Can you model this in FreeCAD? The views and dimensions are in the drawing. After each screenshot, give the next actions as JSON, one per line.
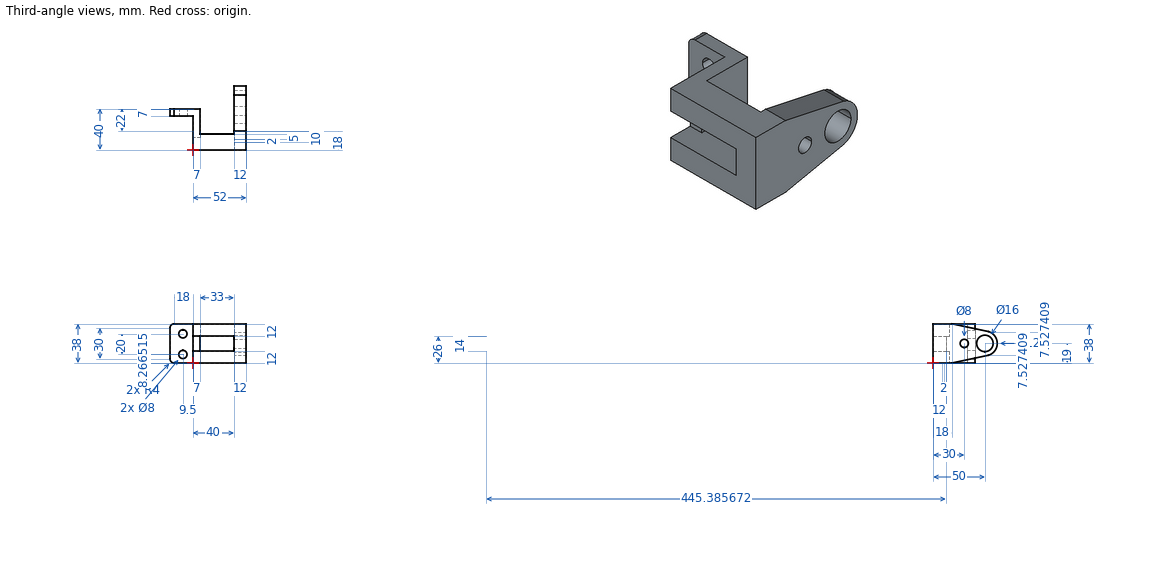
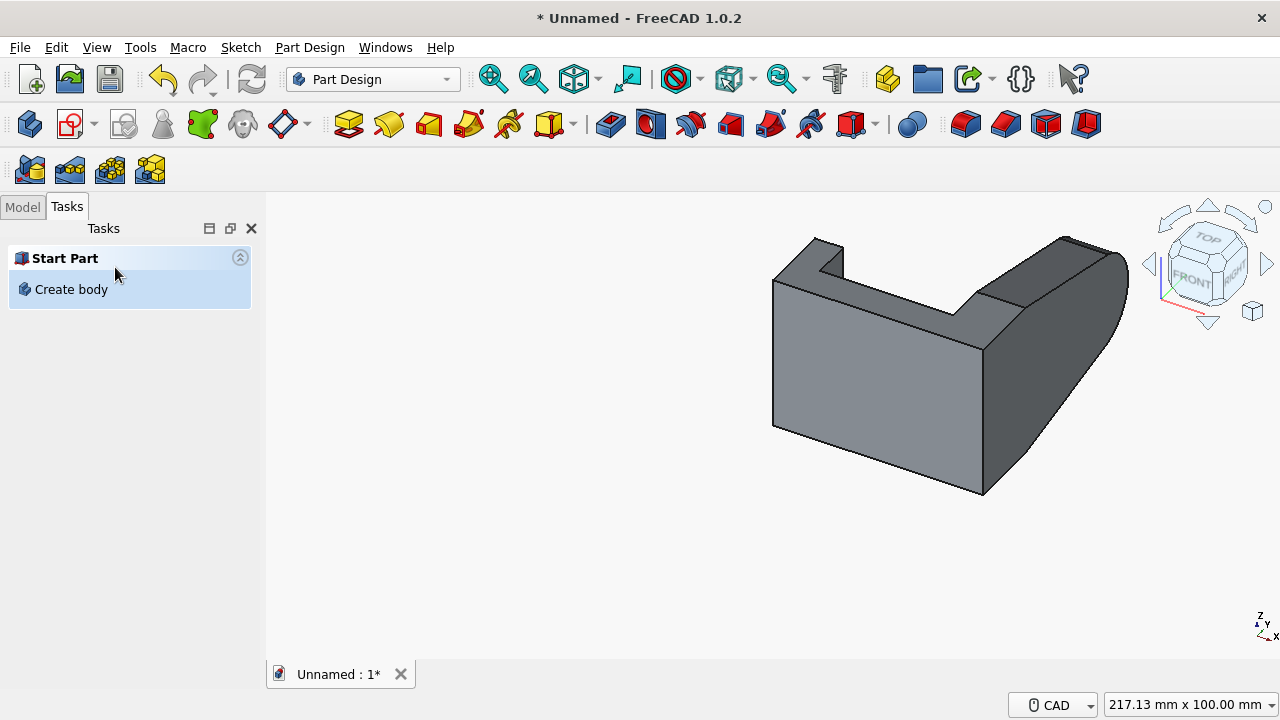
{"action": "left_click", "coordinate": [494, 80]}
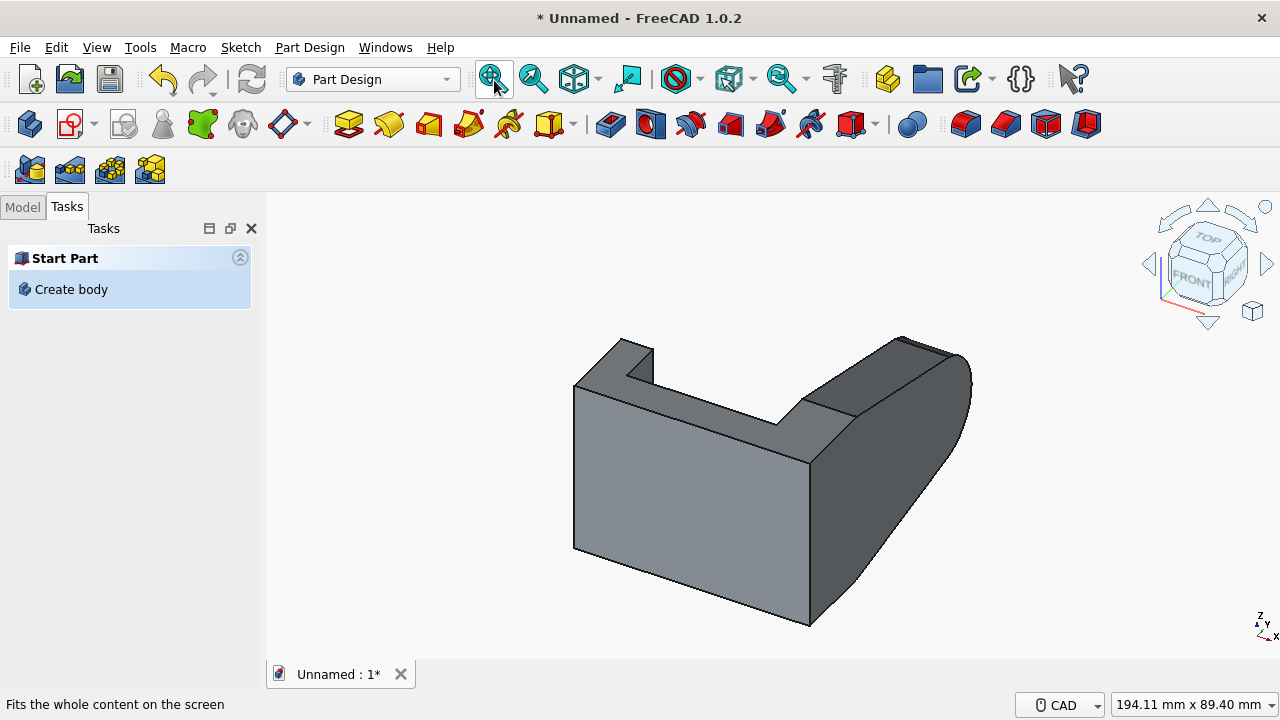
{"action": "left_click", "coordinate": [70, 124]}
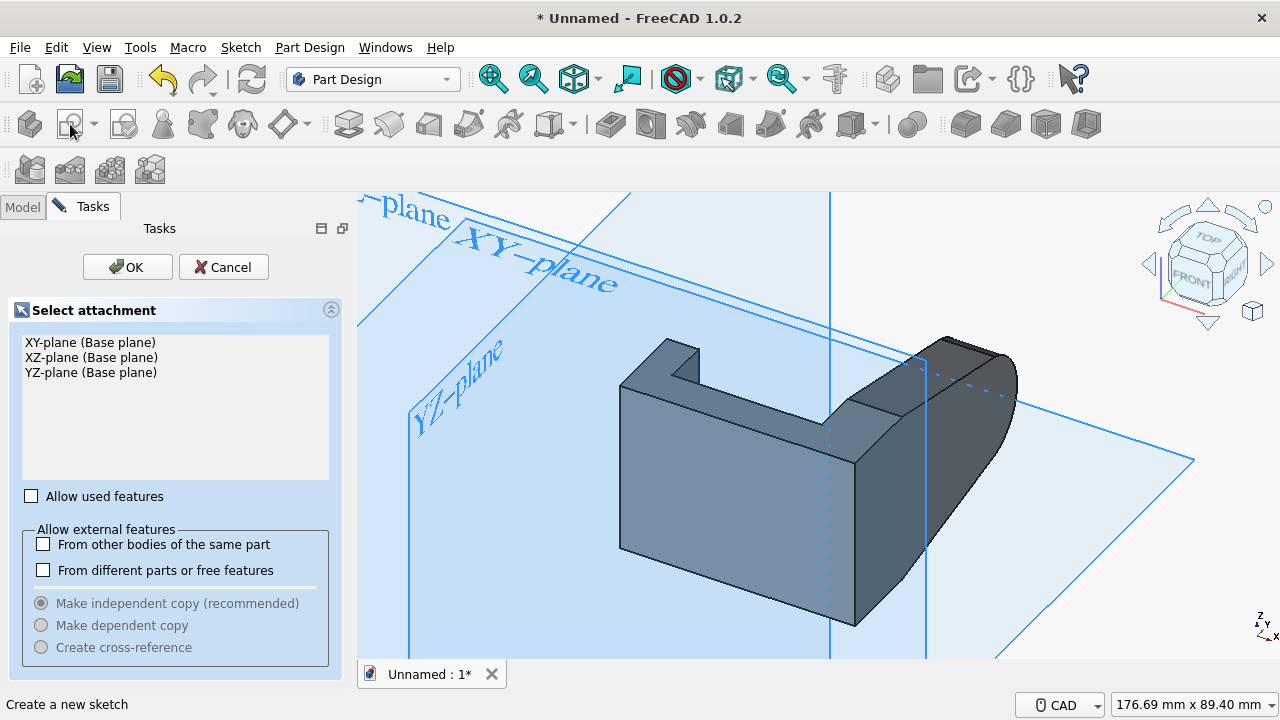
{"action": "left_click", "coordinate": [82, 372]}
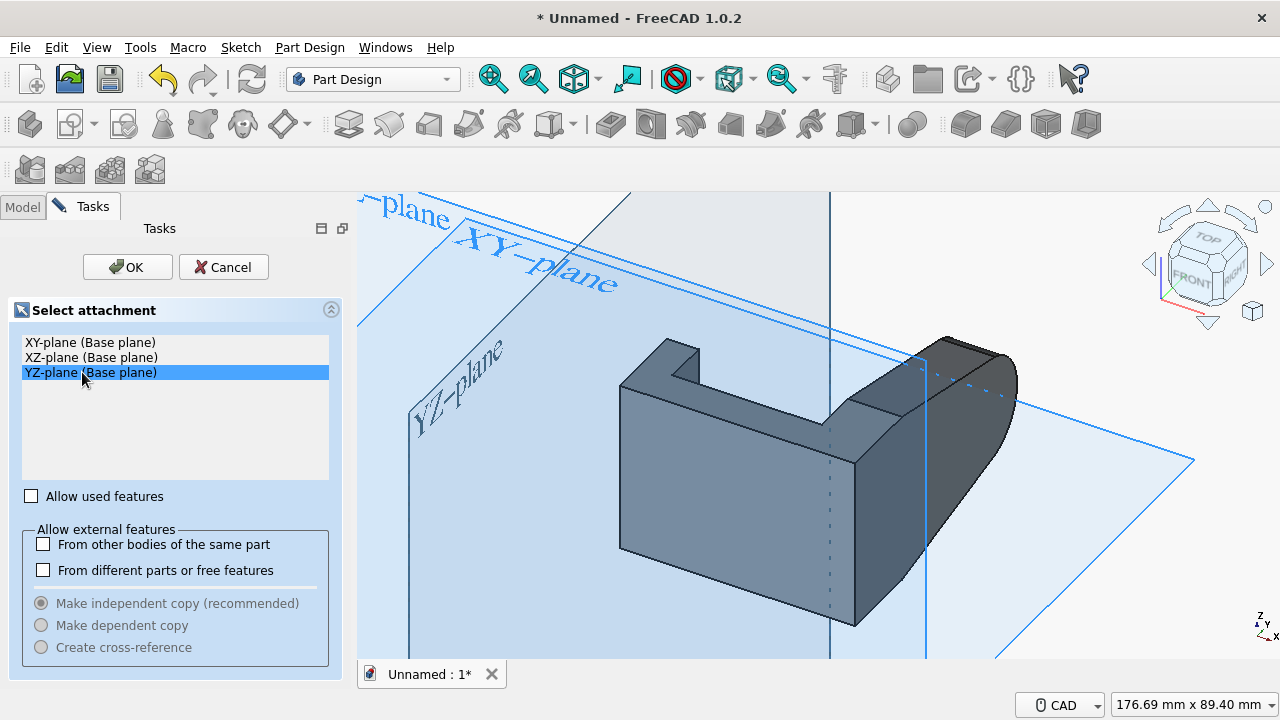
{"action": "left_click", "coordinate": [128, 267]}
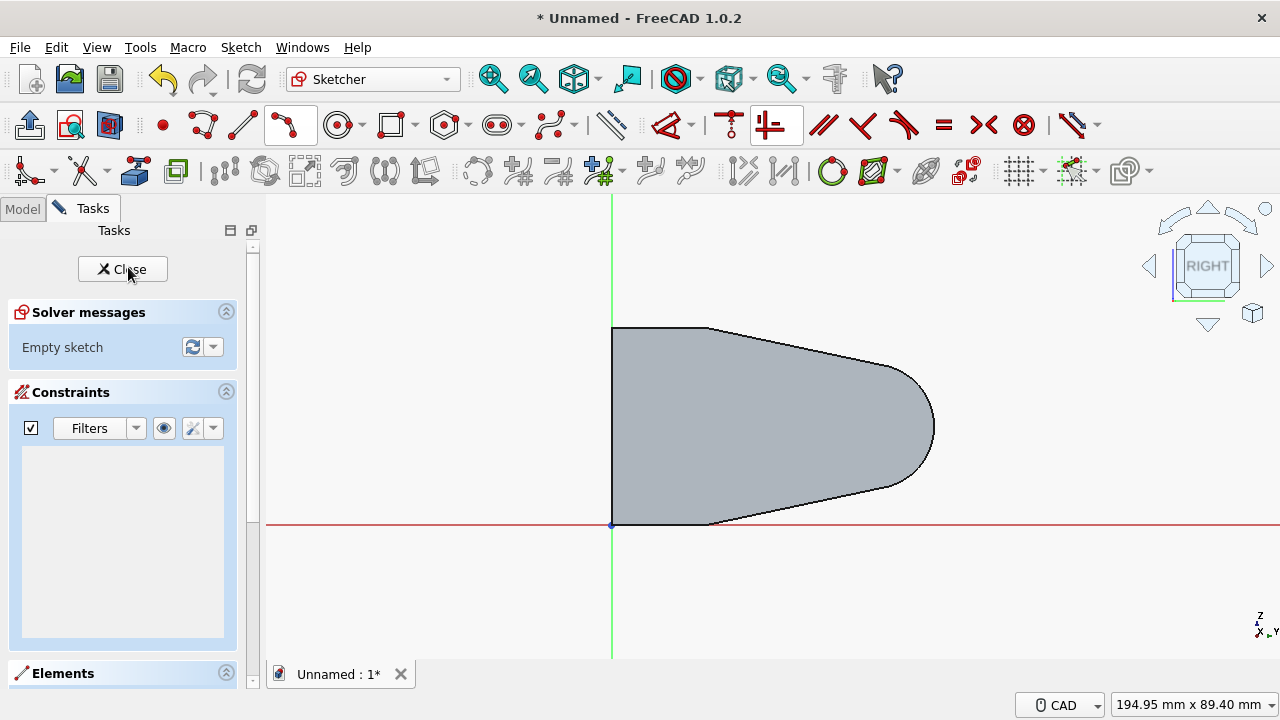
{"action": "left_click", "coordinate": [110, 126]}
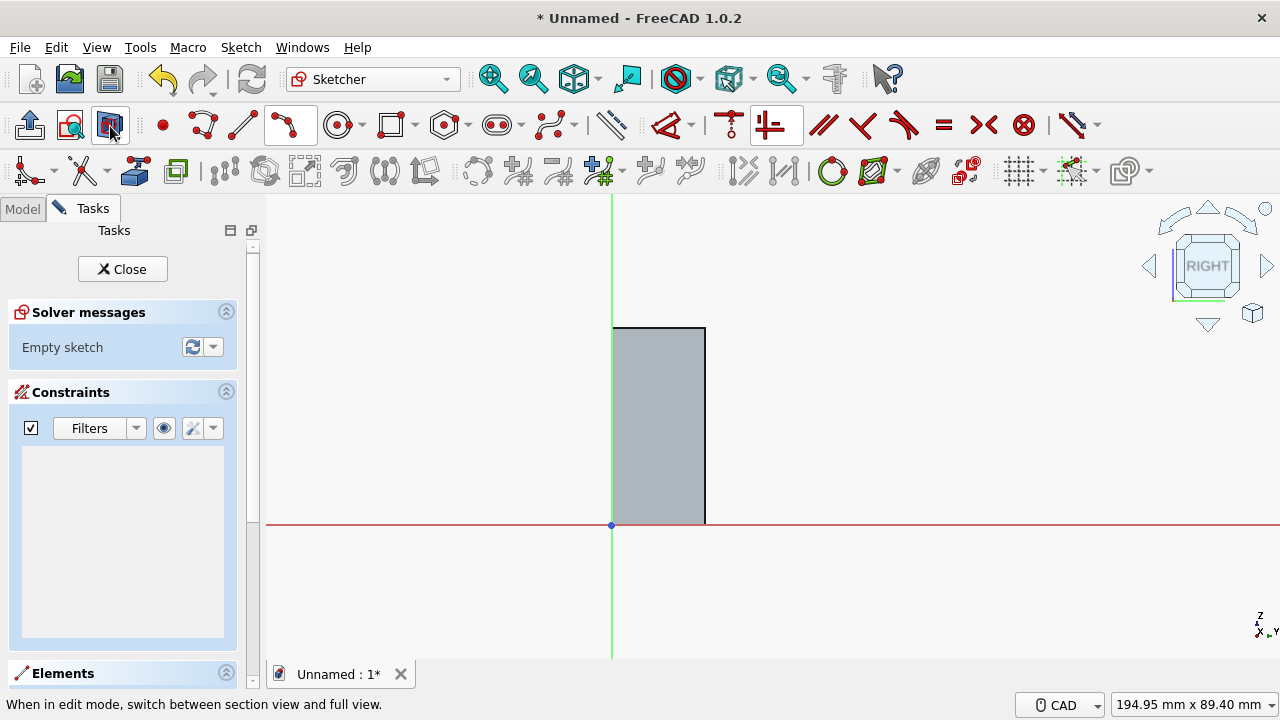
{"action": "scroll", "coordinate": [1094, 416], "scroll_direction": "down", "scroll_amount": 7}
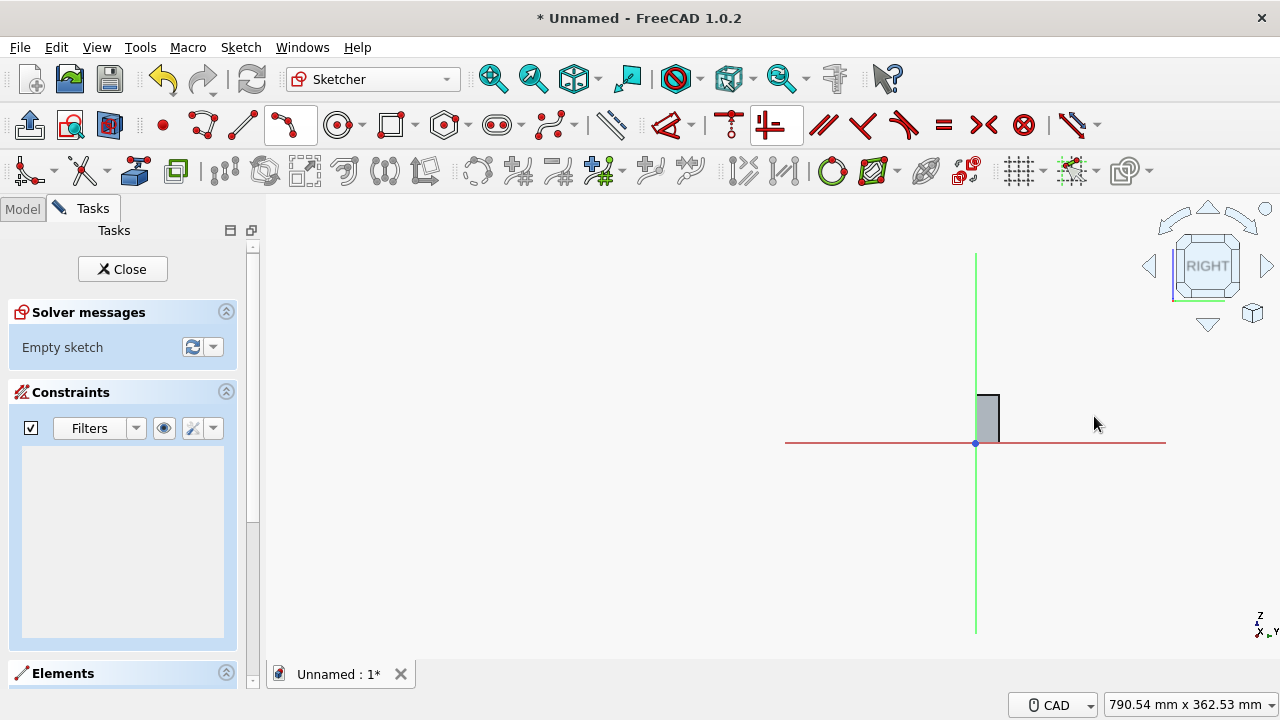
{"action": "left_click", "coordinate": [392, 126]}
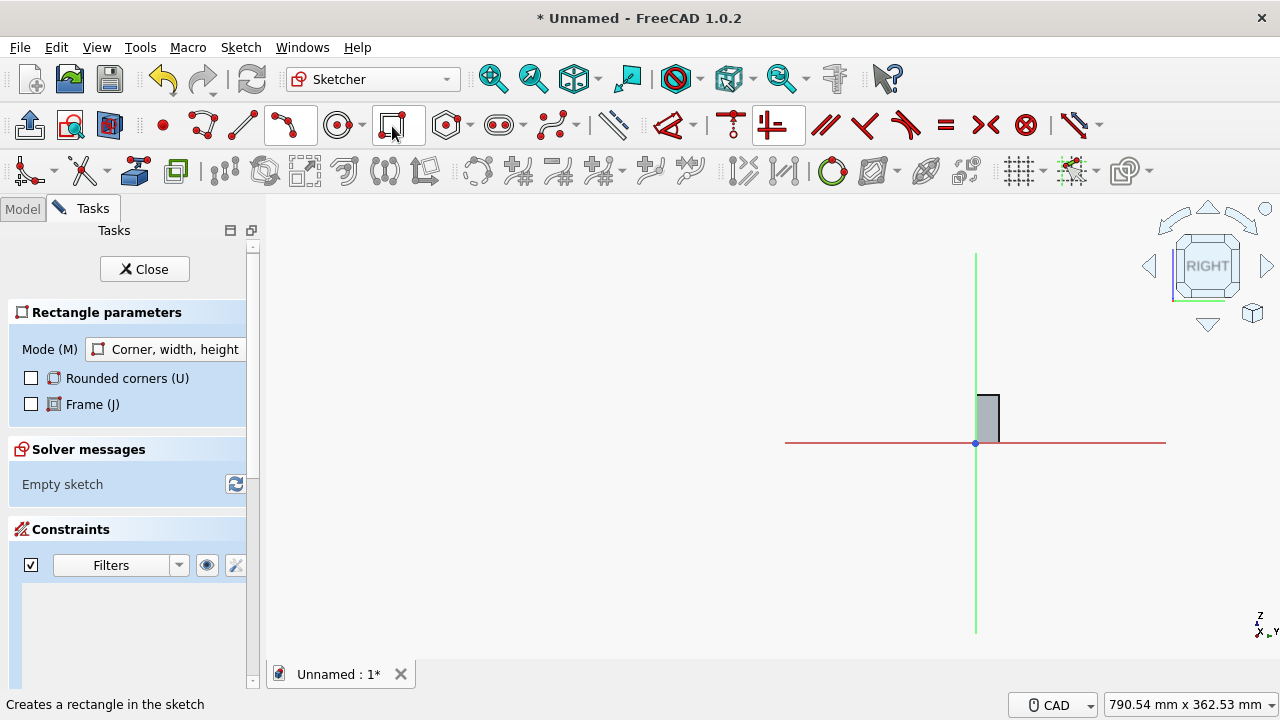
{"action": "left_click", "coordinate": [420, 410]}
{"action": "left_click", "coordinate": [991, 428]}
{"action": "key", "text": "Escape"}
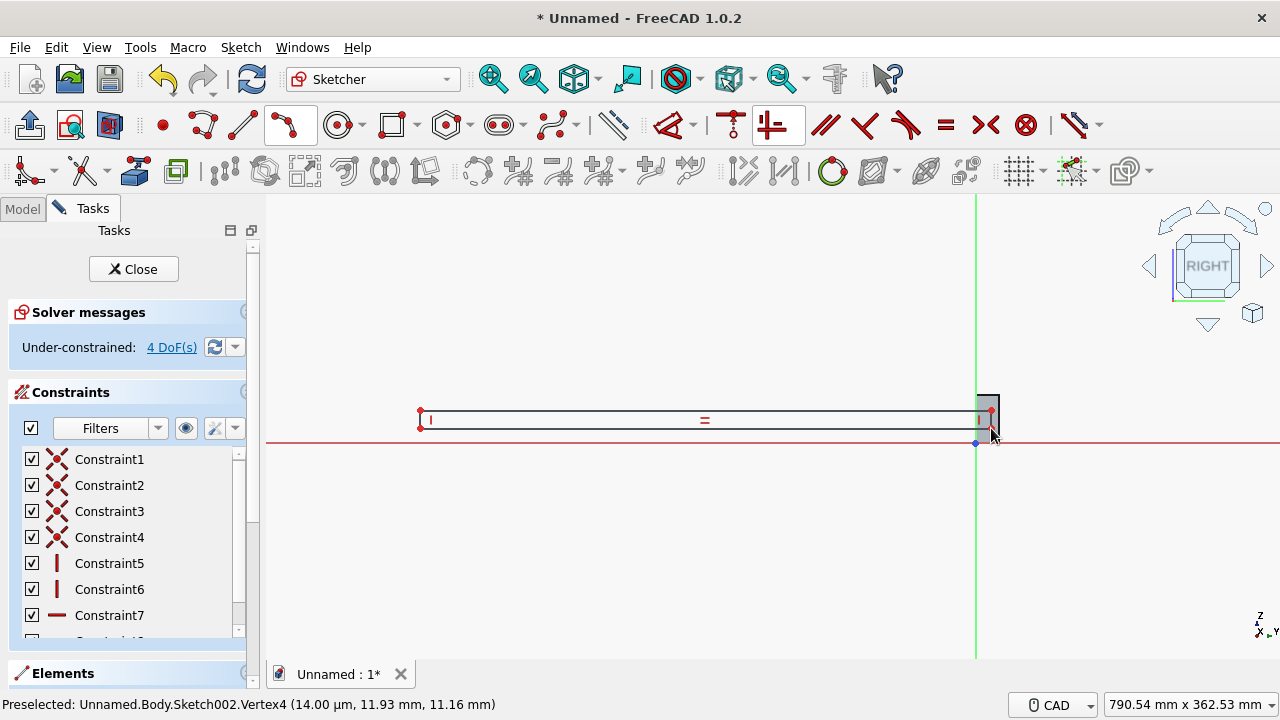
{"action": "left_click", "coordinate": [668, 126]}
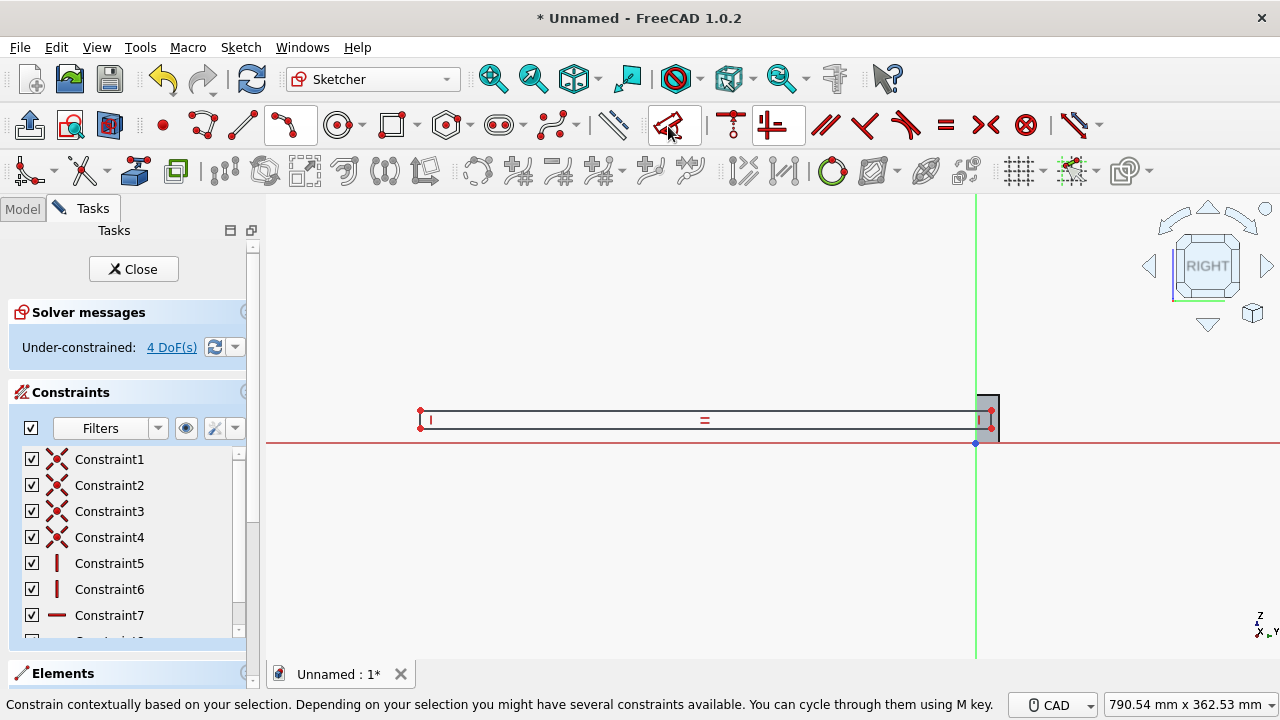
{"action": "scroll", "coordinate": [420, 420], "scroll_direction": "up", "scroll_amount": 4}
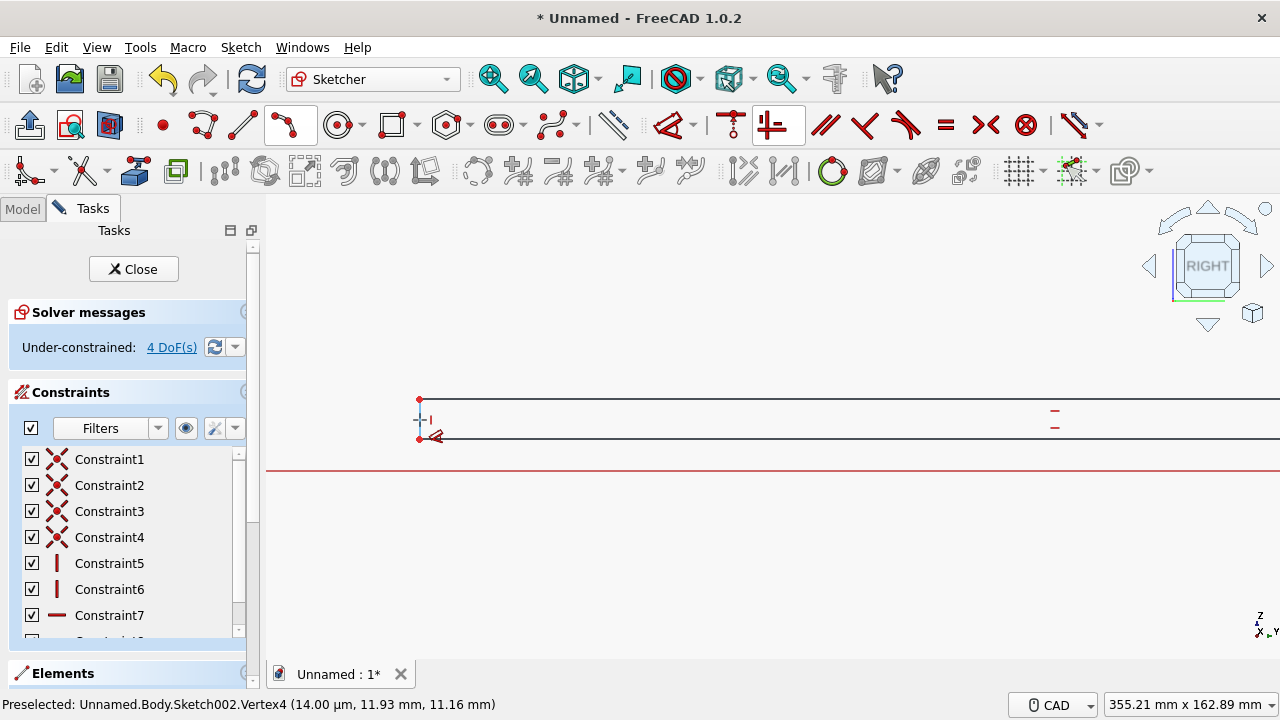
{"action": "left_click", "coordinate": [420, 419]}
{"action": "left_click", "coordinate": [386, 419]}